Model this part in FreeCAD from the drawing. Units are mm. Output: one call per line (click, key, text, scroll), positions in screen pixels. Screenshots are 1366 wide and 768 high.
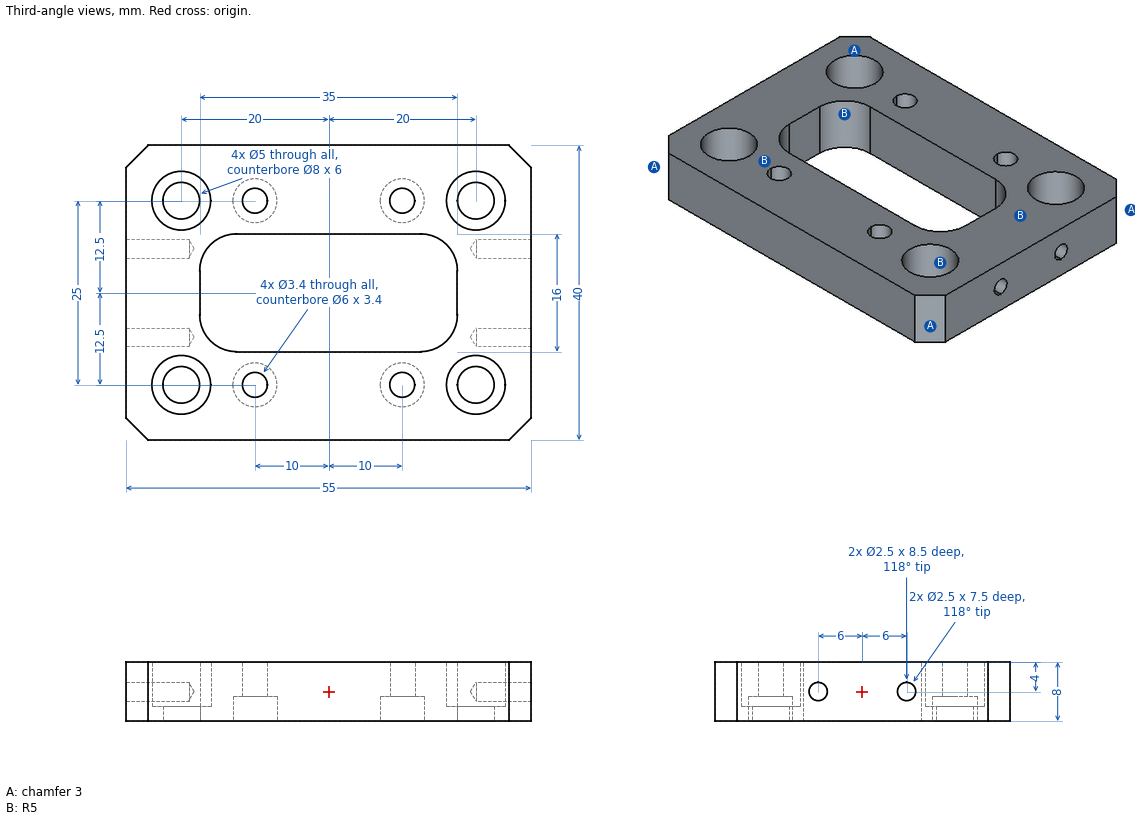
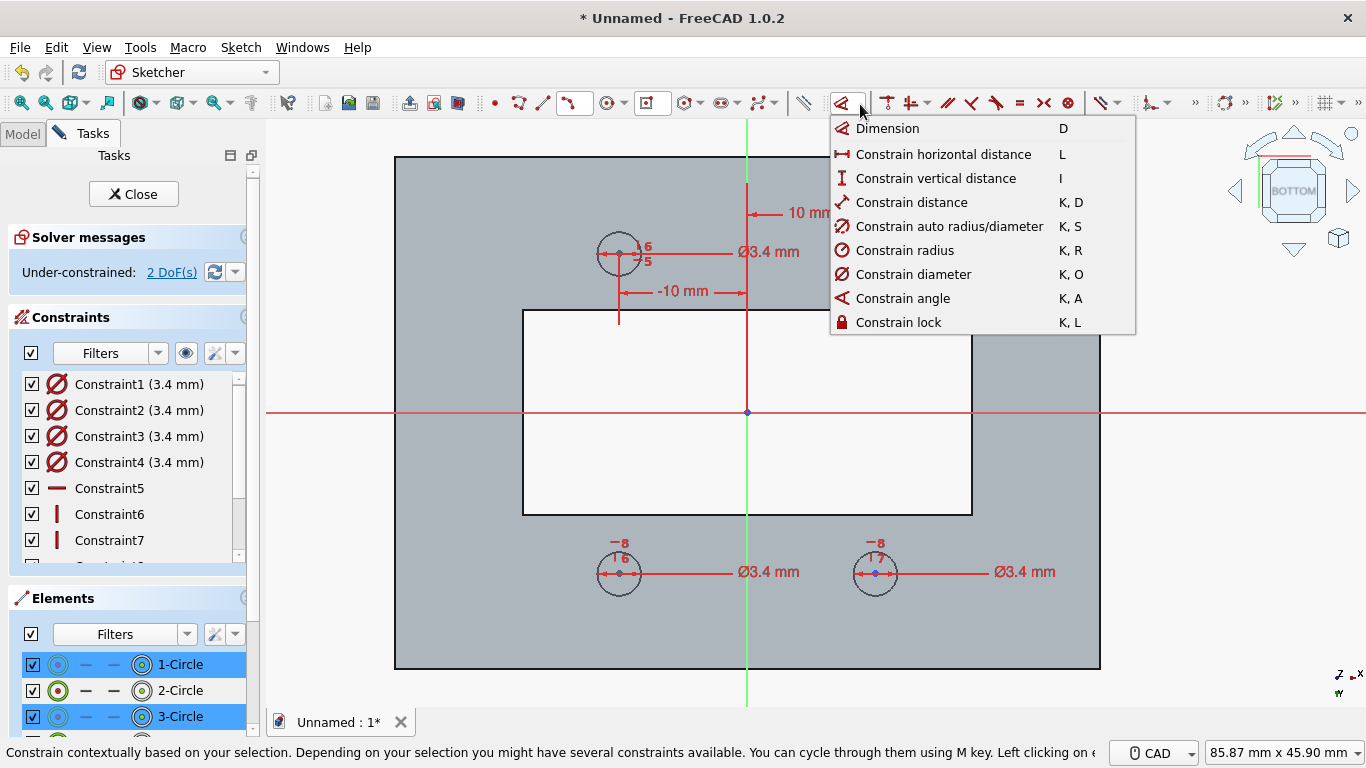
click(983, 178)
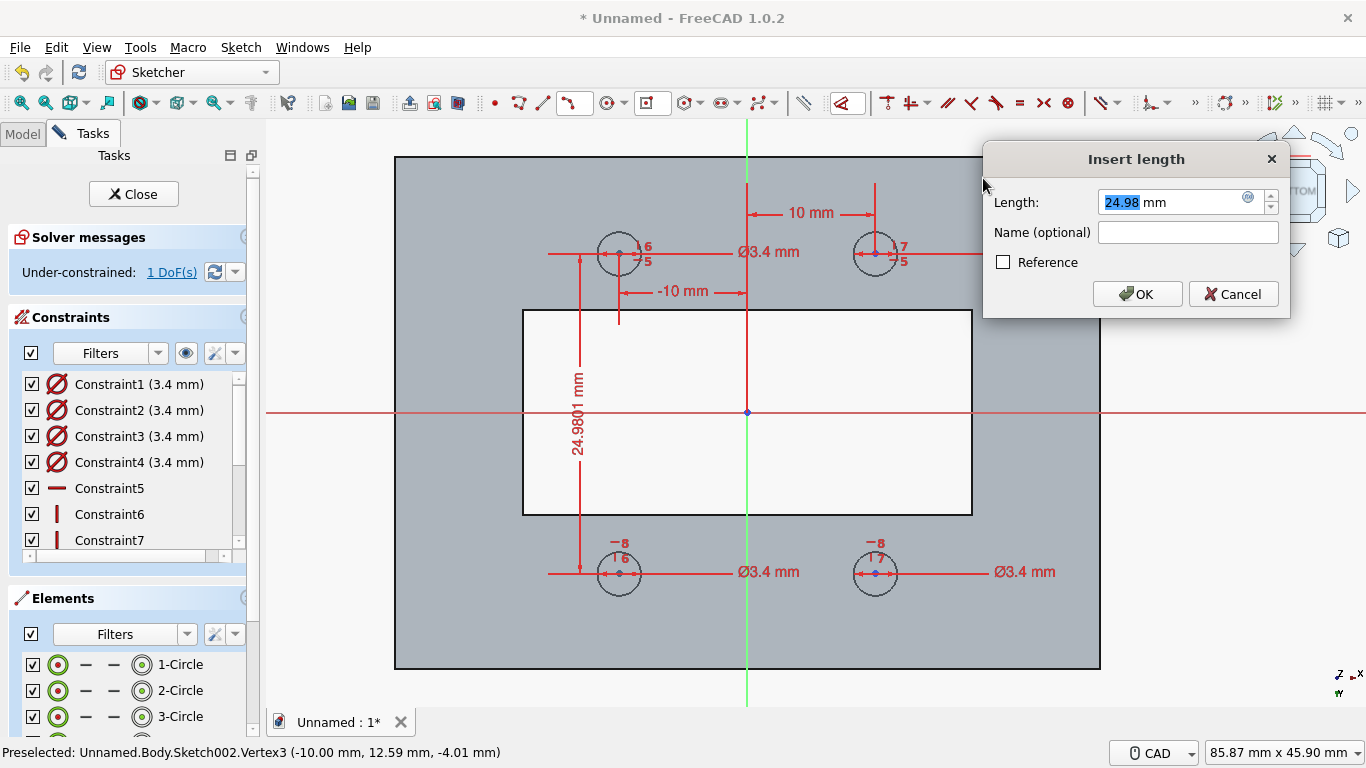
text(25)
key(Return)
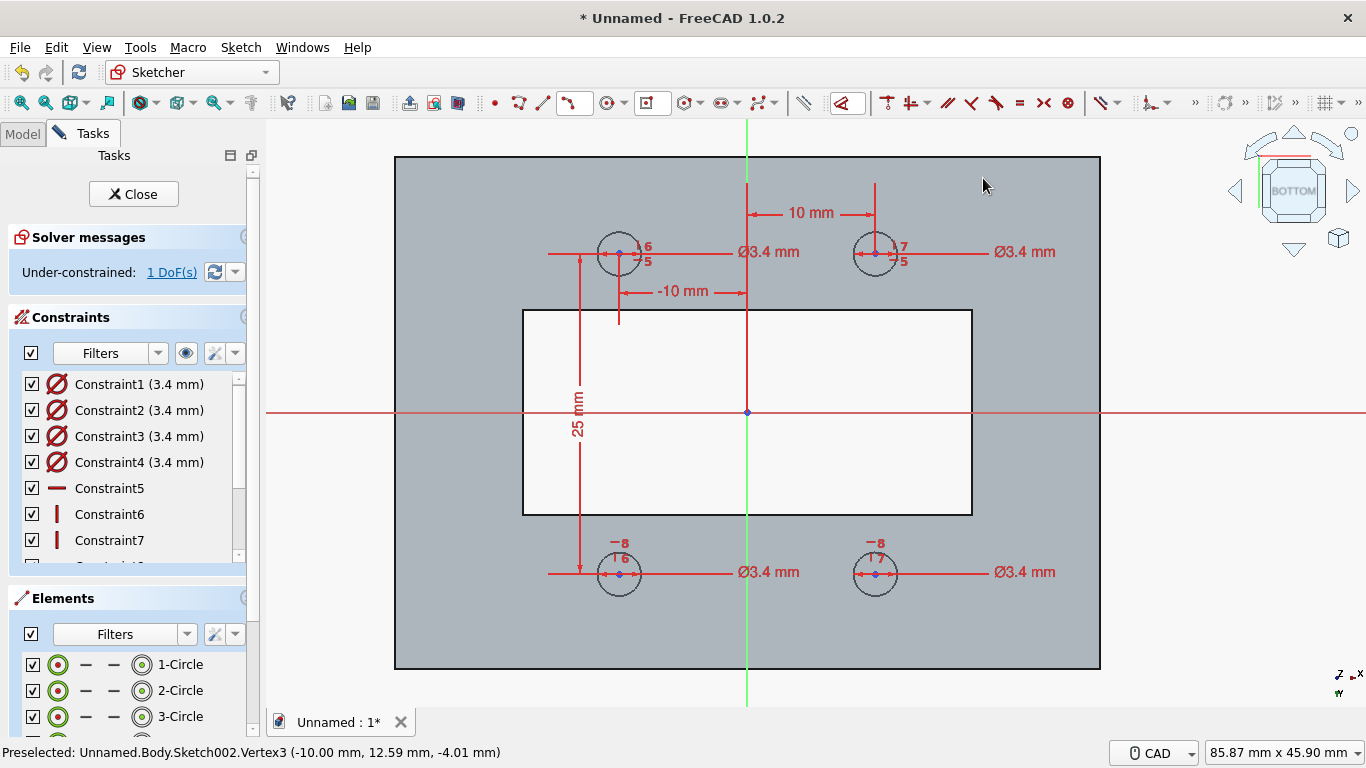
click(619, 254)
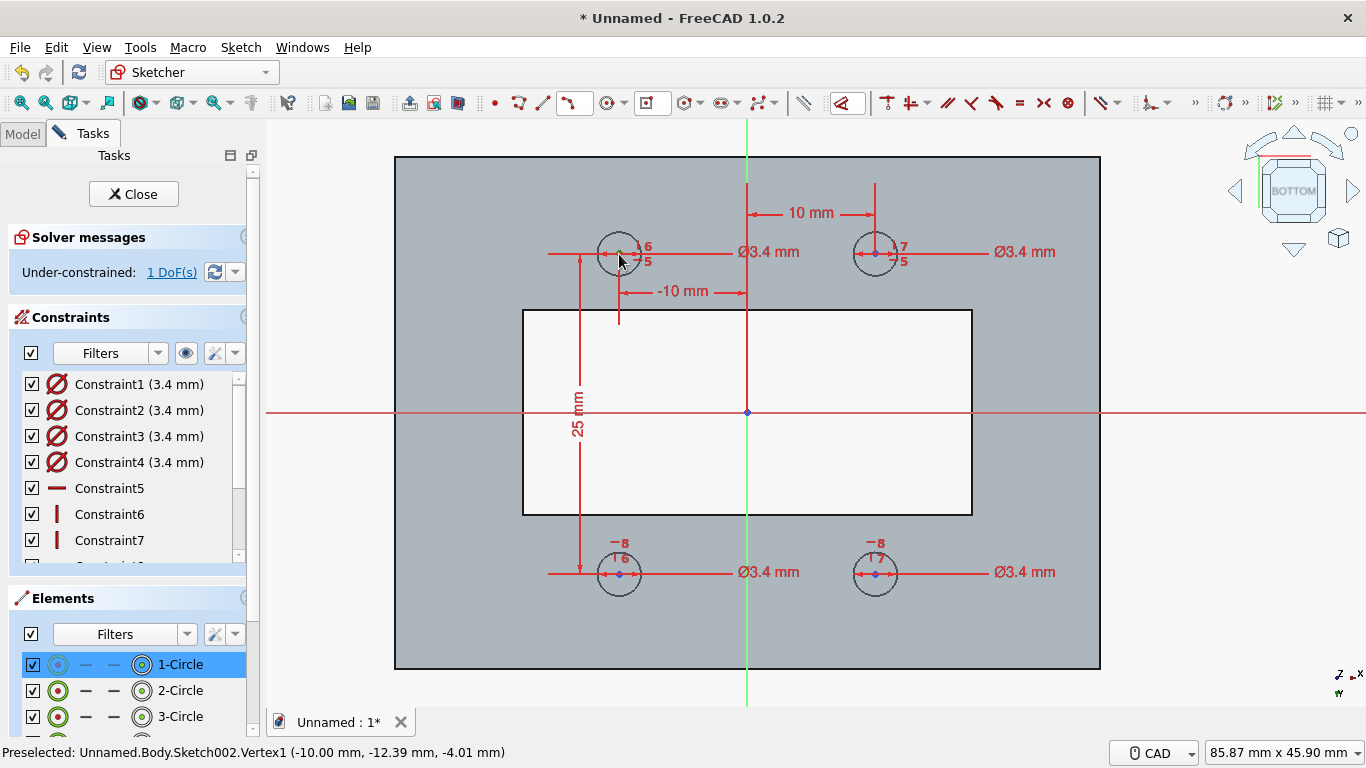
click(860, 104)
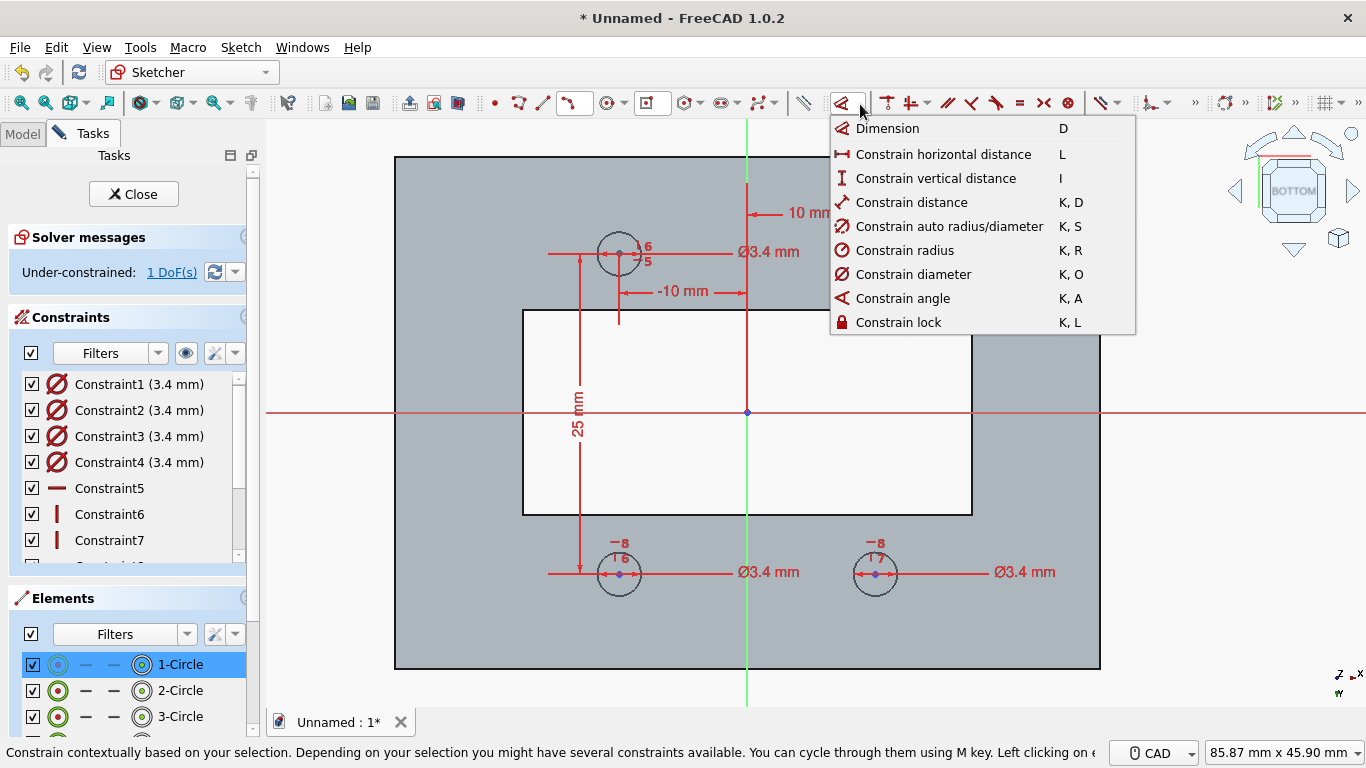
click(983, 178)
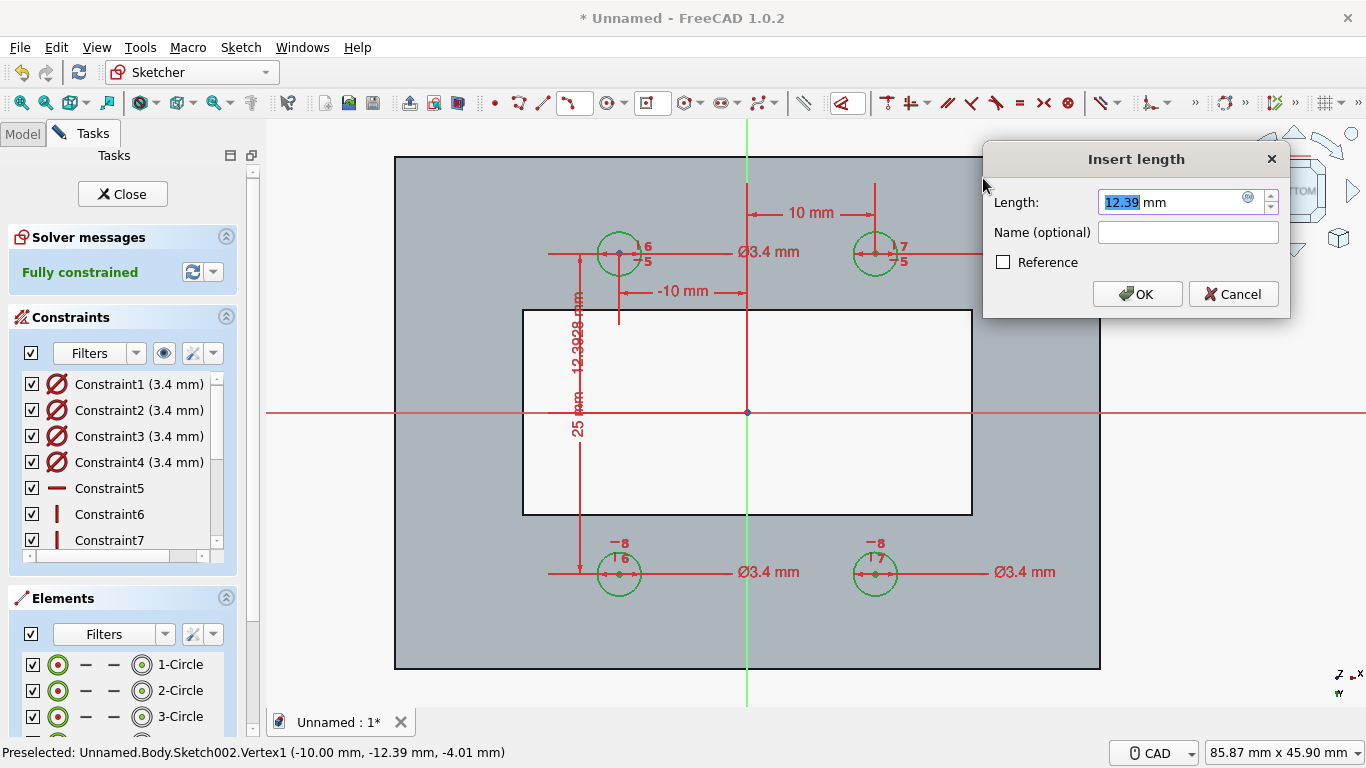
text(12.5)
key(Return)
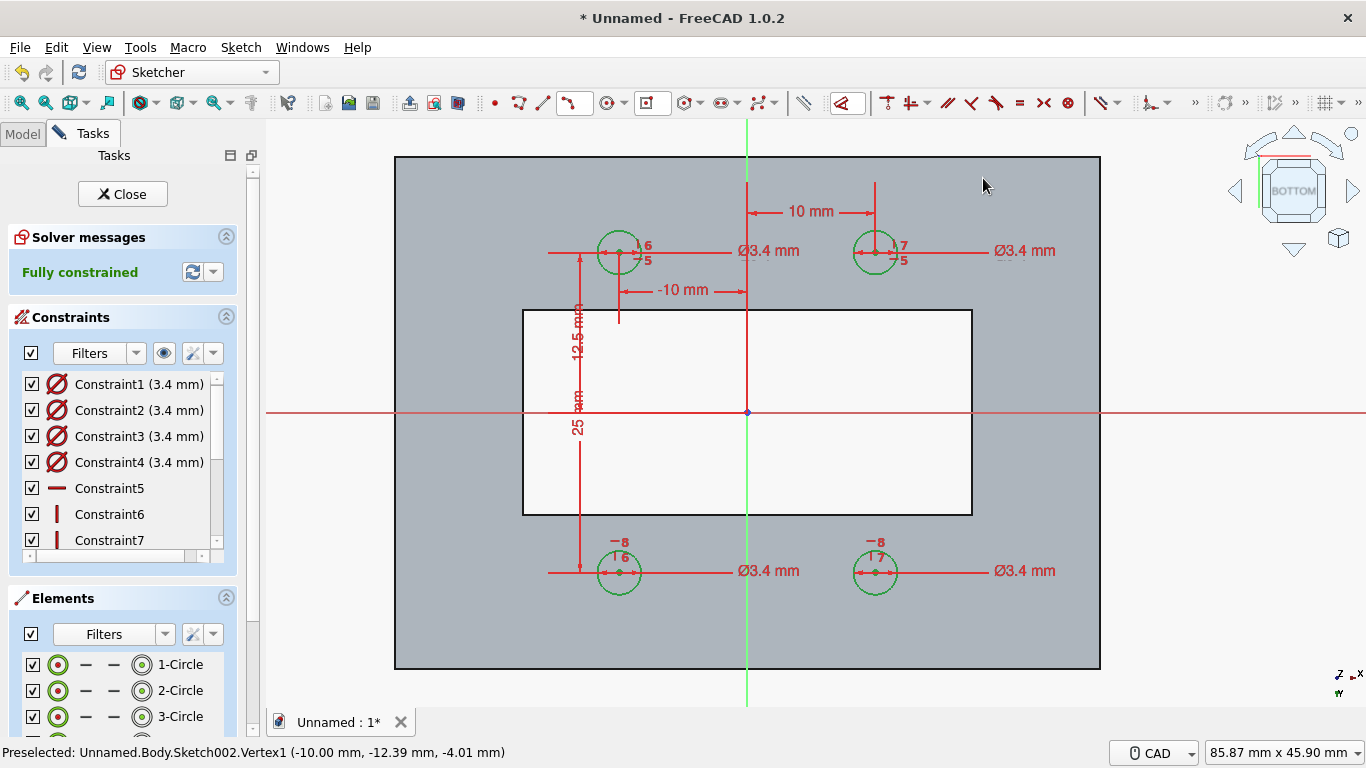
click(123, 194)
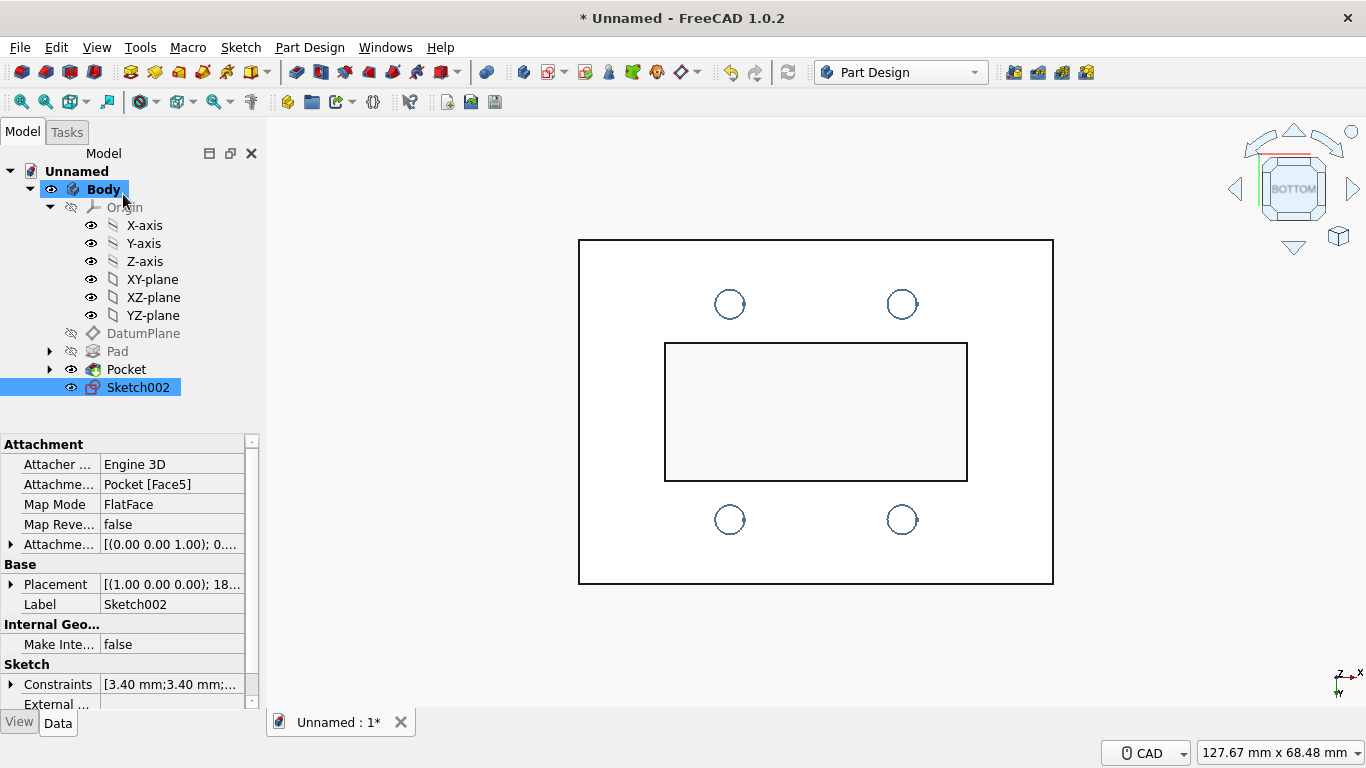
click(322, 72)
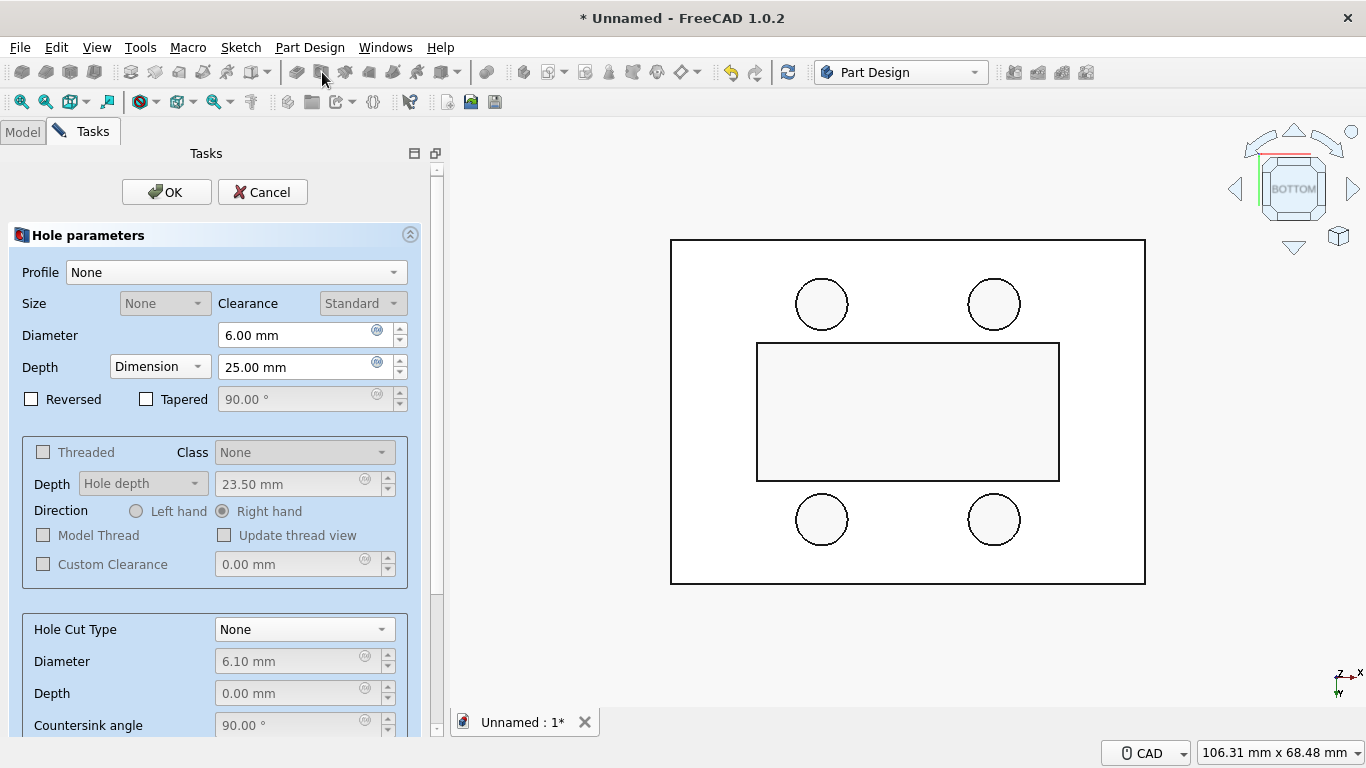
triple_click(305, 335)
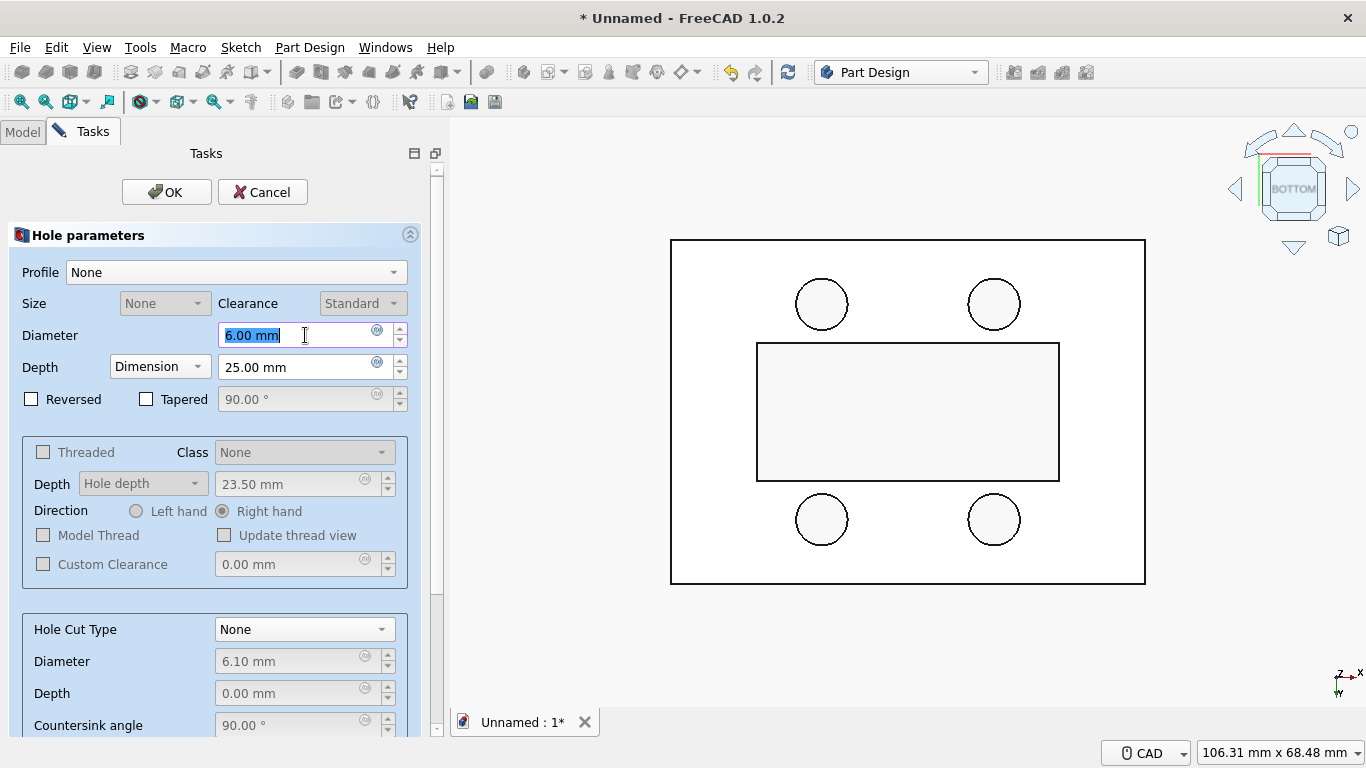
text(3.4)
key(Tab)